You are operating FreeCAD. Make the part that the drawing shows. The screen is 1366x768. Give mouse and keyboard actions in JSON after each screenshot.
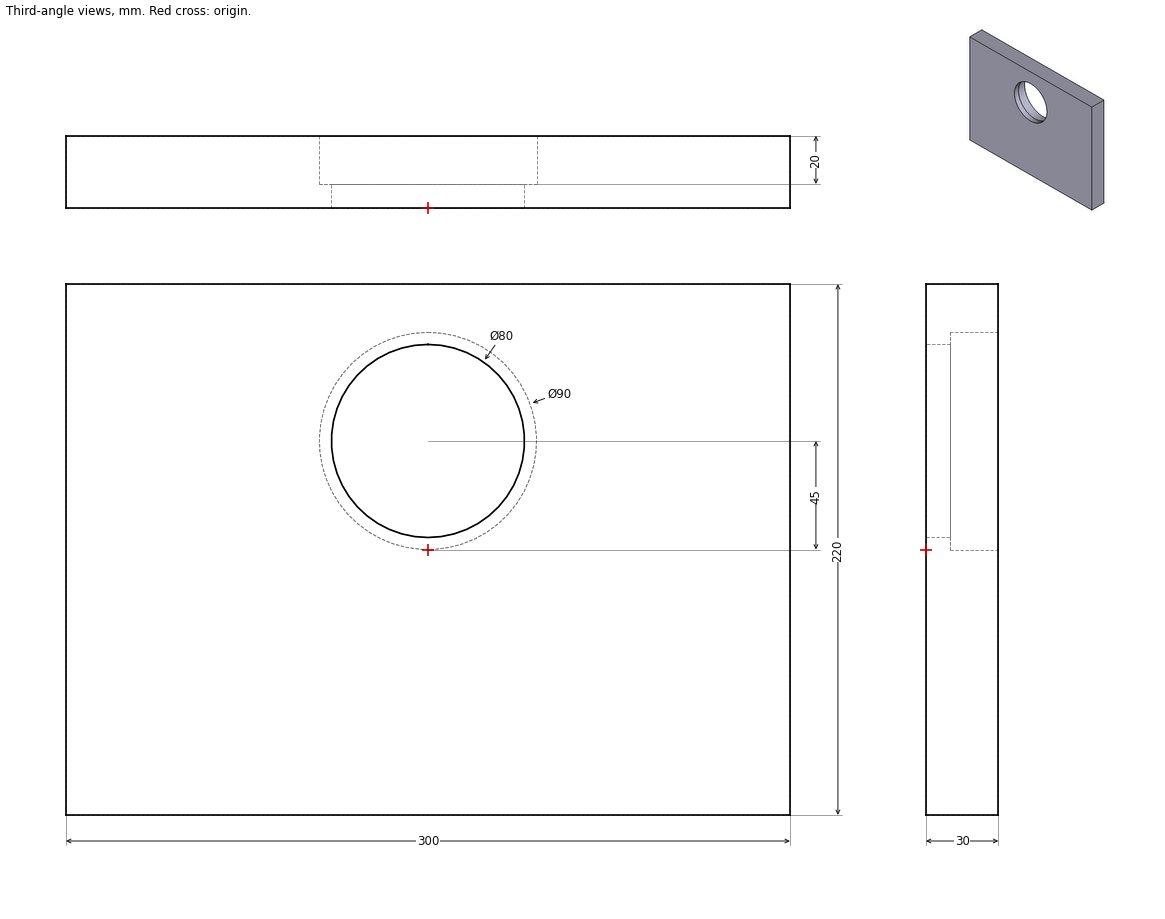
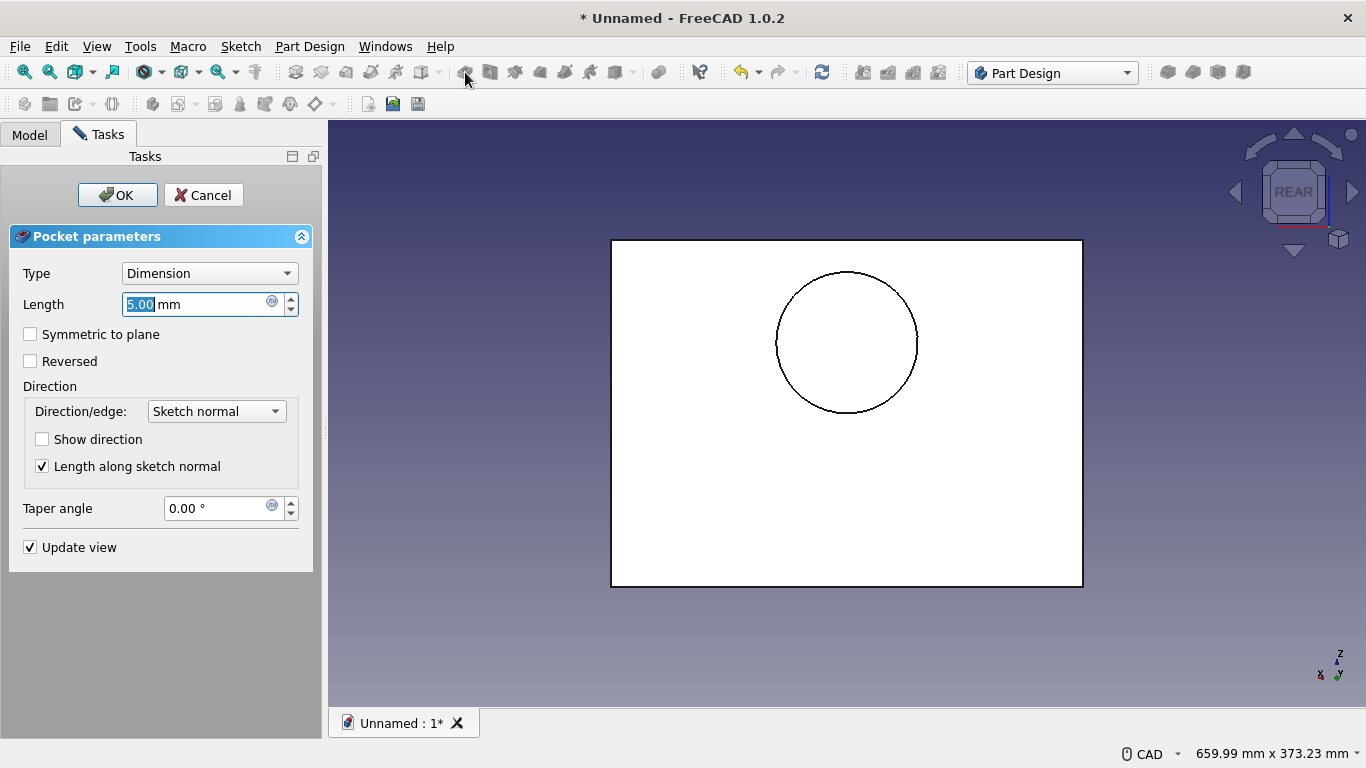
{"action": "left_click", "coordinate": [210, 274]}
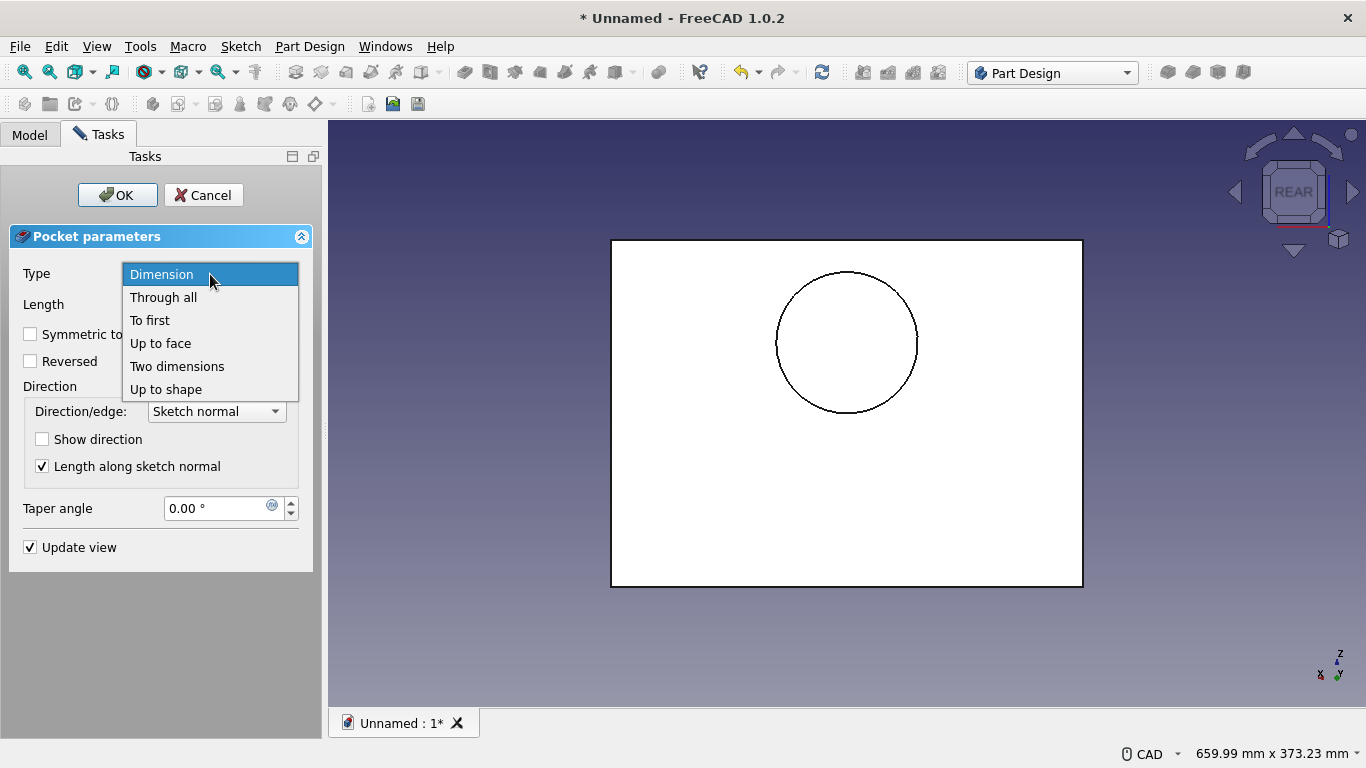
{"action": "left_click", "coordinate": [208, 298]}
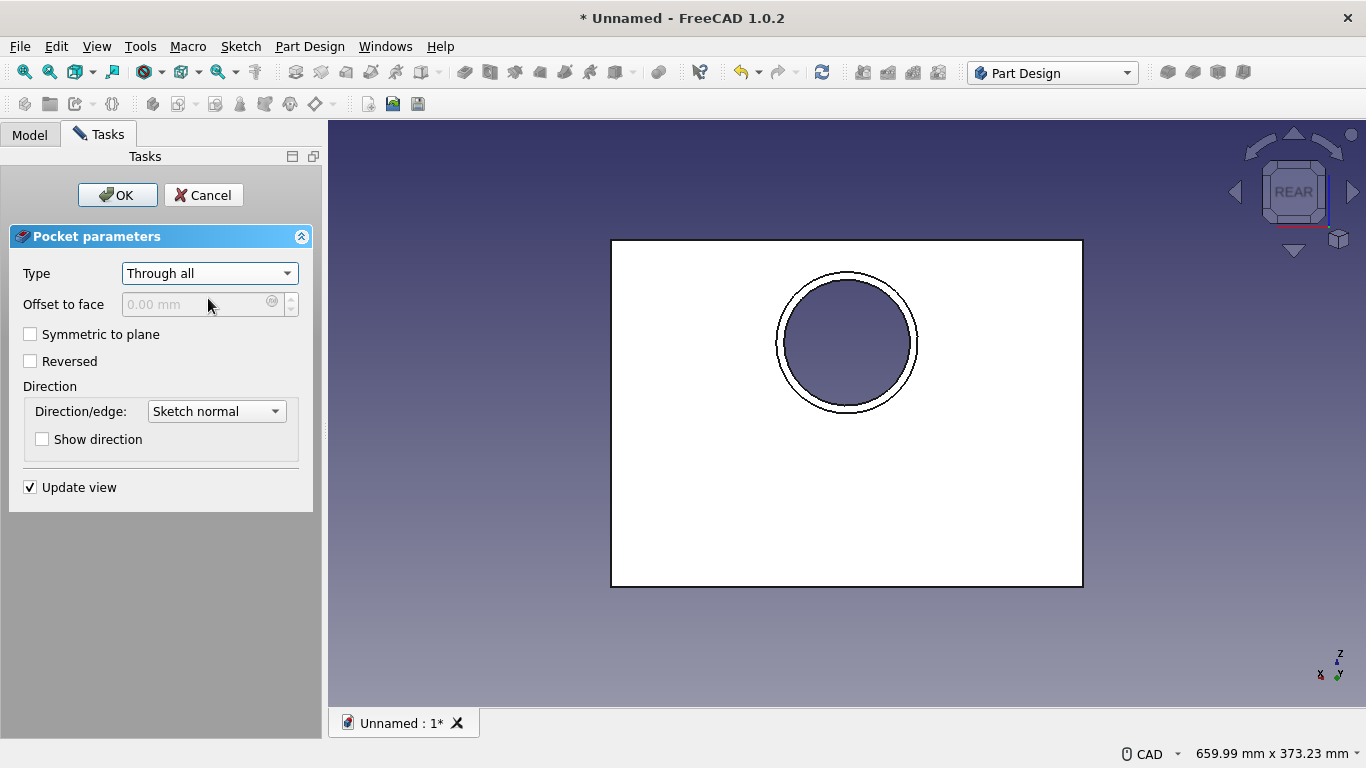
{"action": "left_click", "coordinate": [118, 195]}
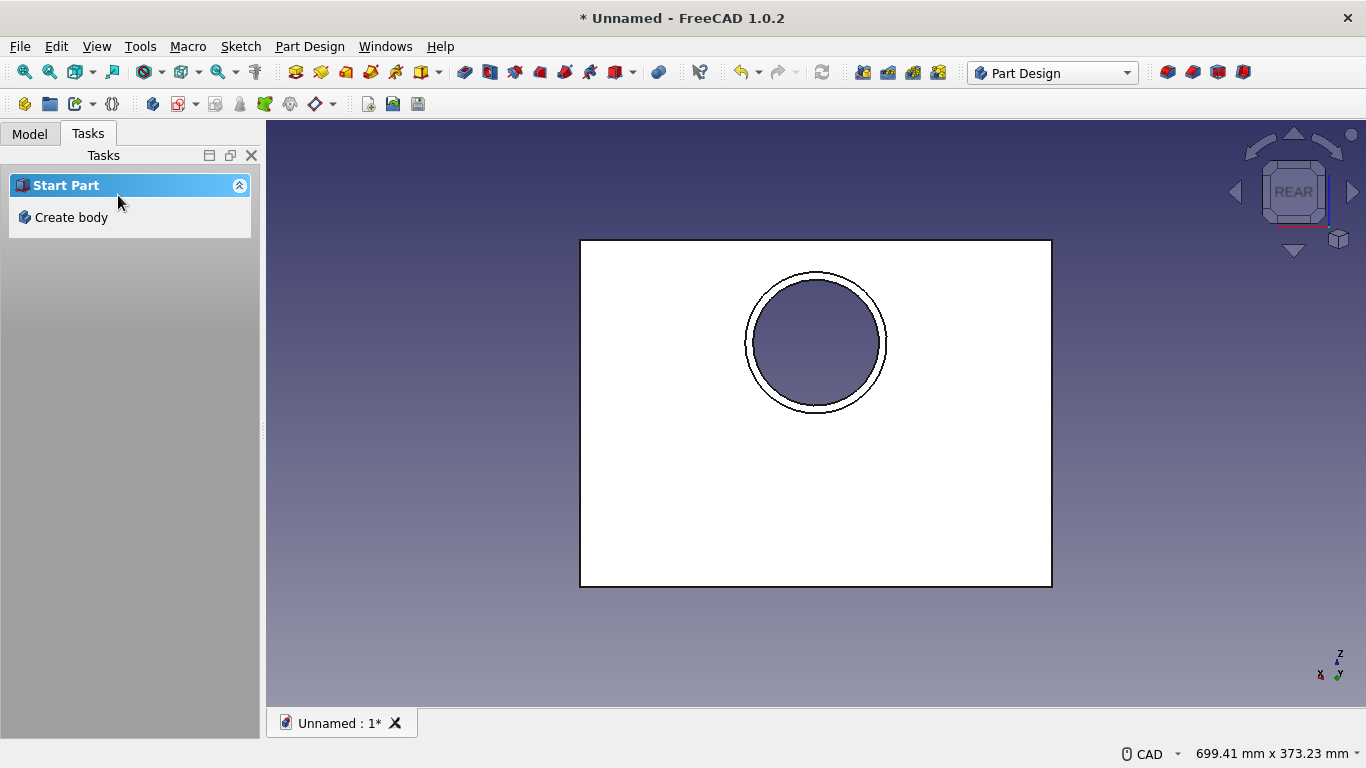
{"action": "key", "text": "0"}